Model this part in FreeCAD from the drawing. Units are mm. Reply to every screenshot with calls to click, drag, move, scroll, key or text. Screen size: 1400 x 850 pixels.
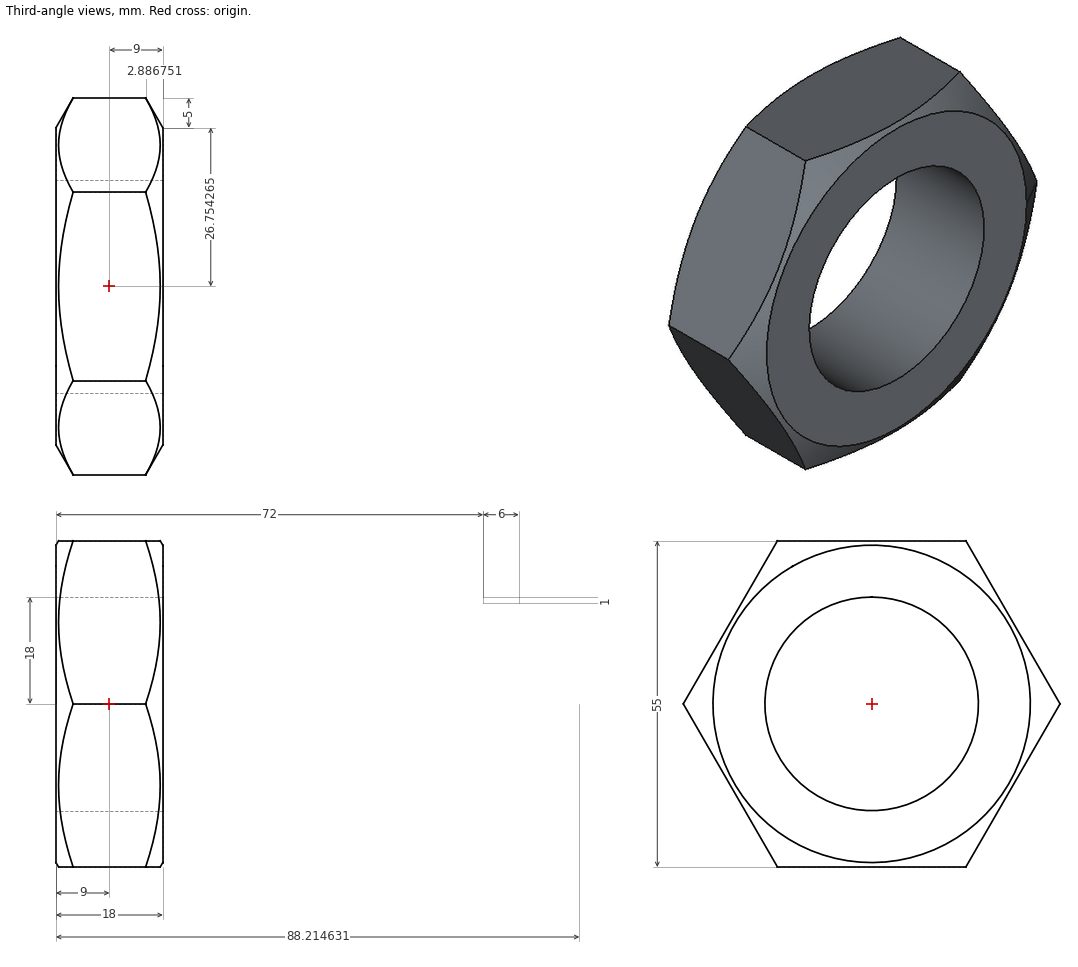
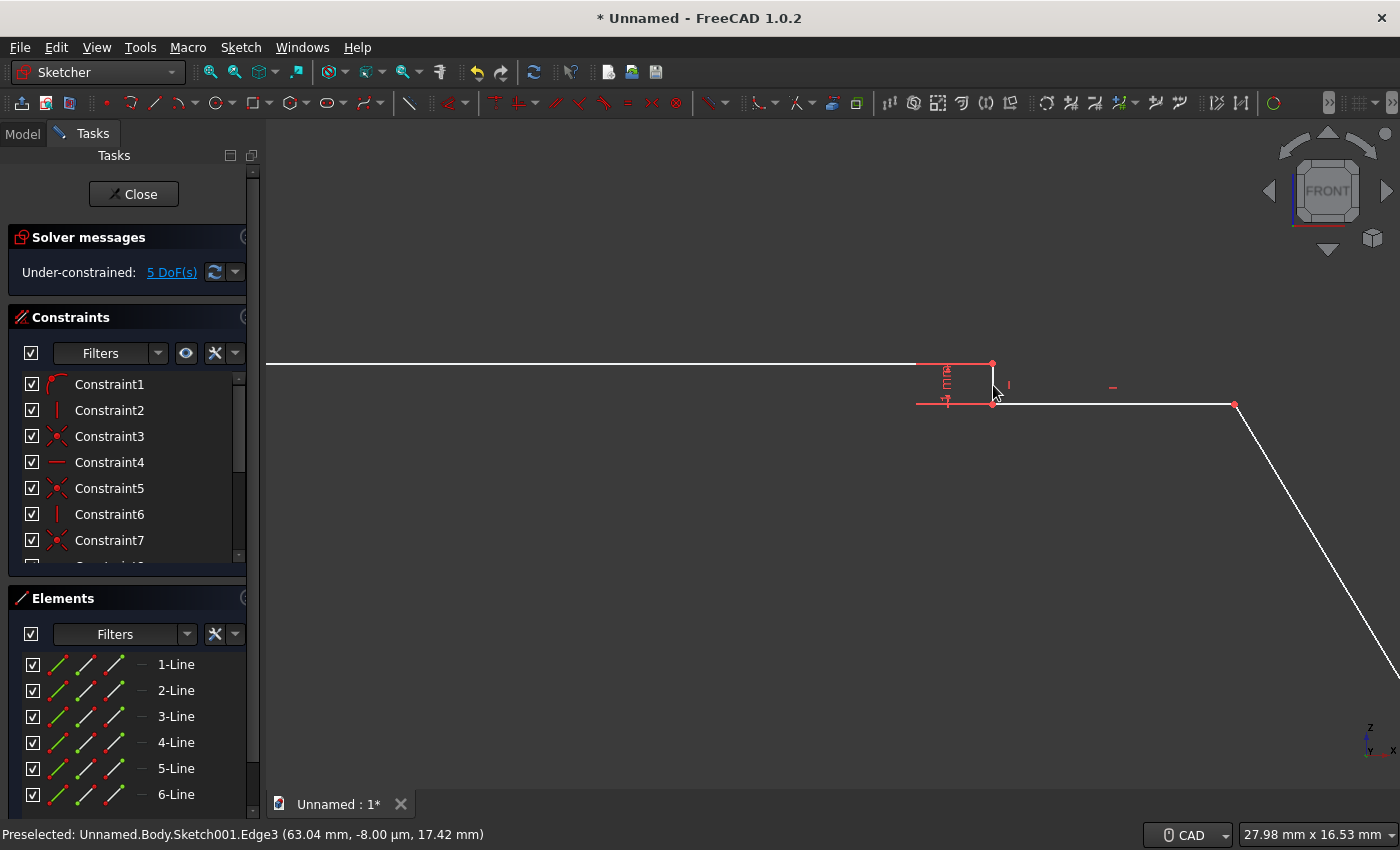
scroll(993, 385, down, 8)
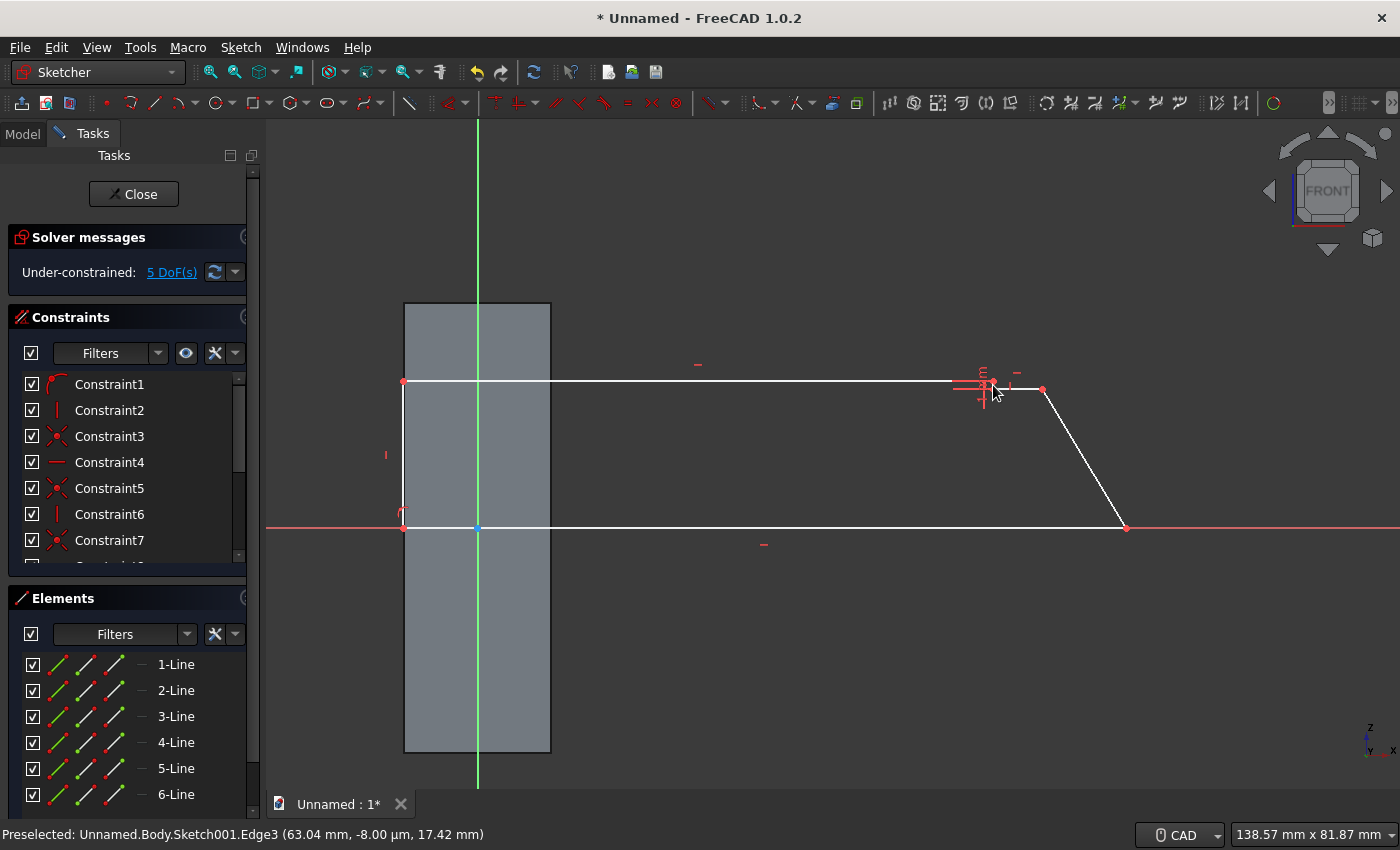
click(1028, 389)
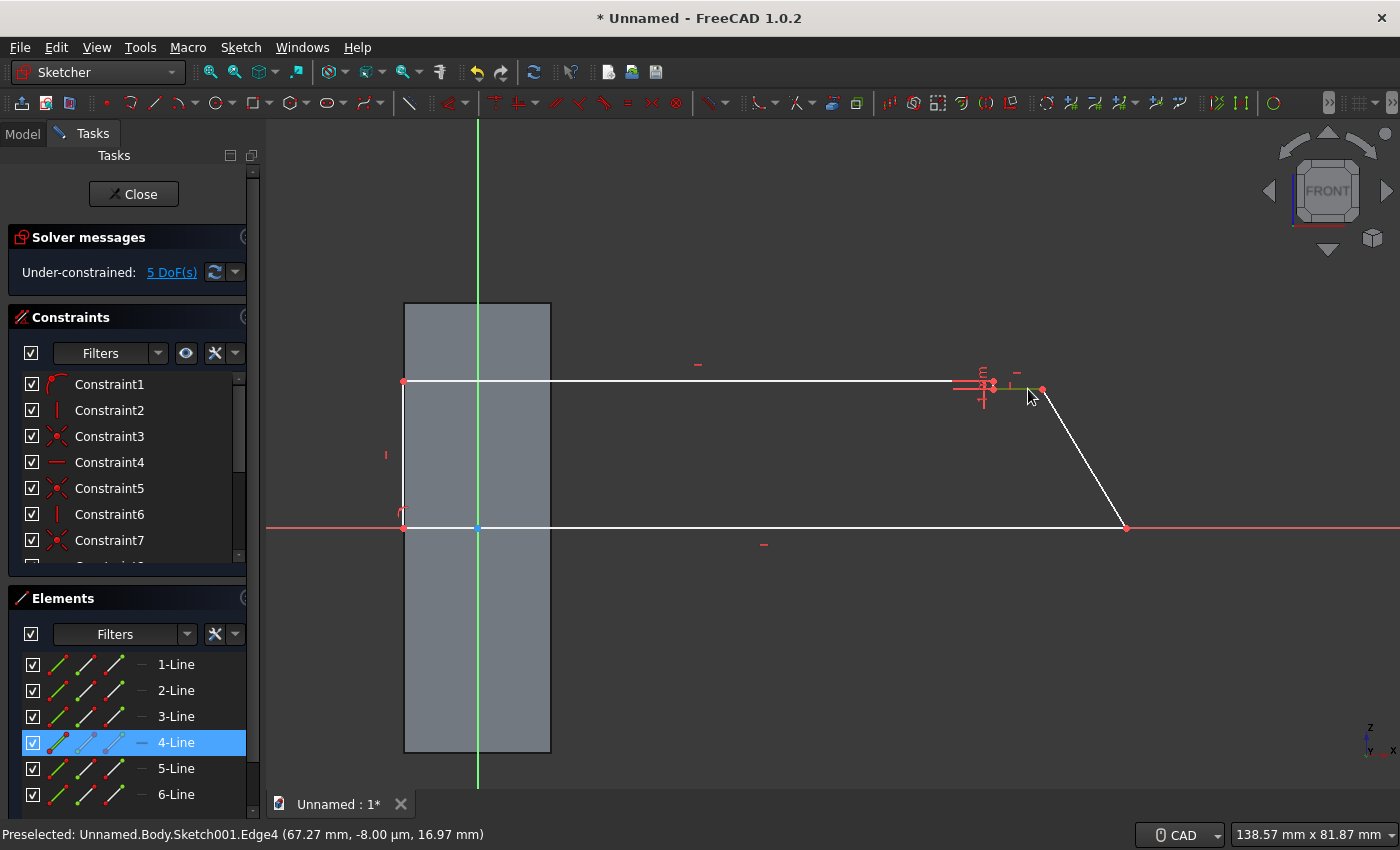
key(l)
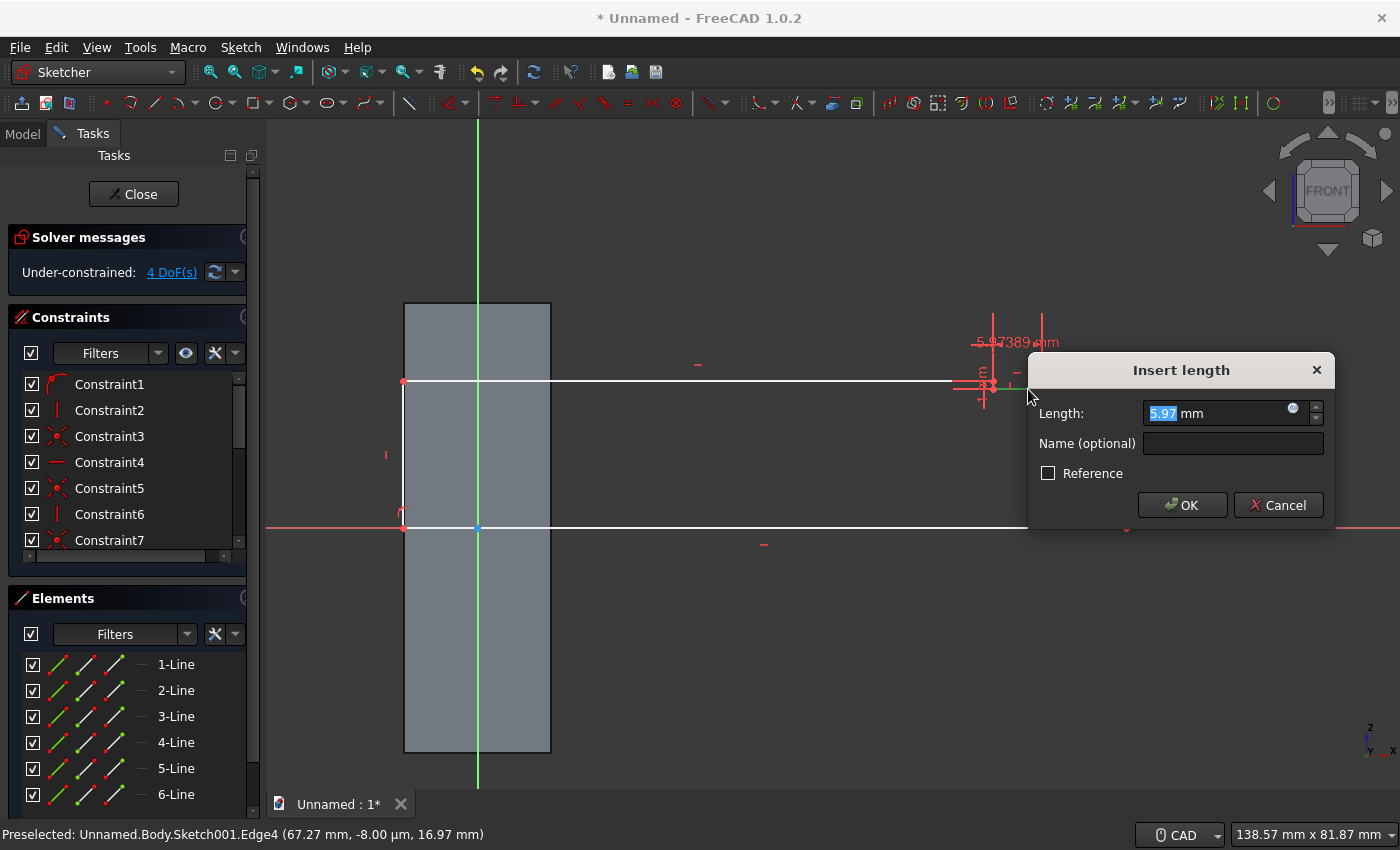
text(6)
key(Return)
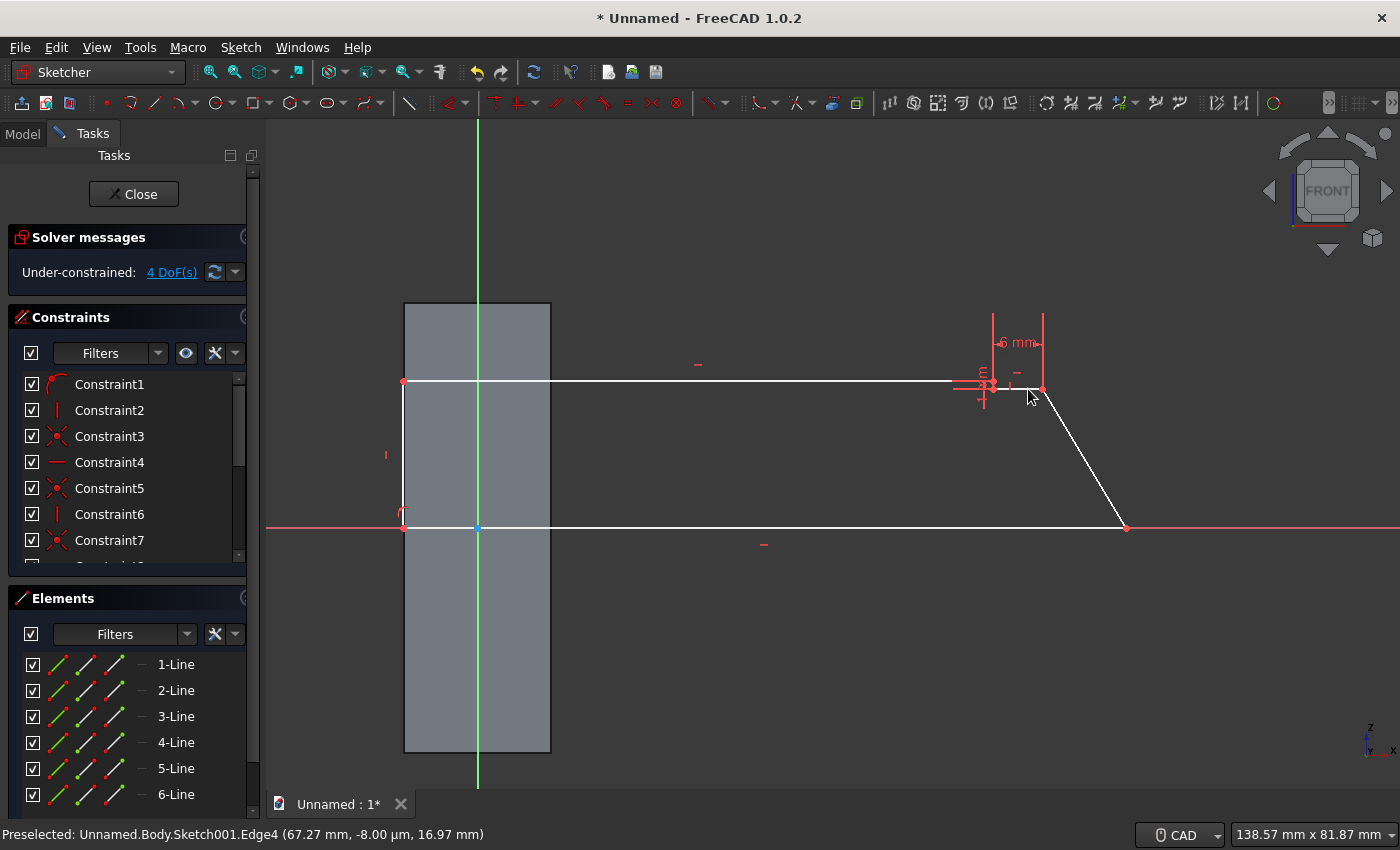
click(403, 484)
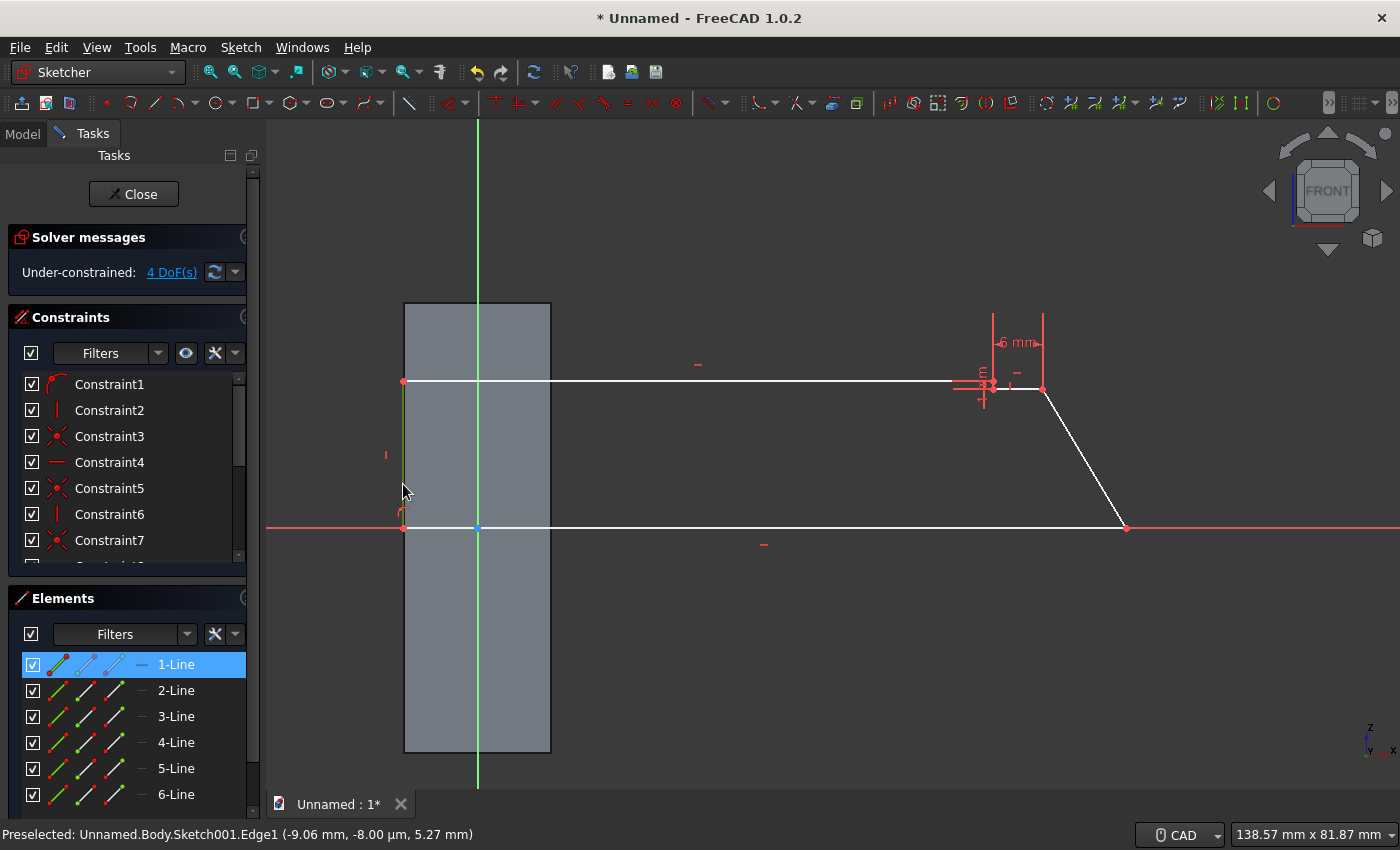
key(i)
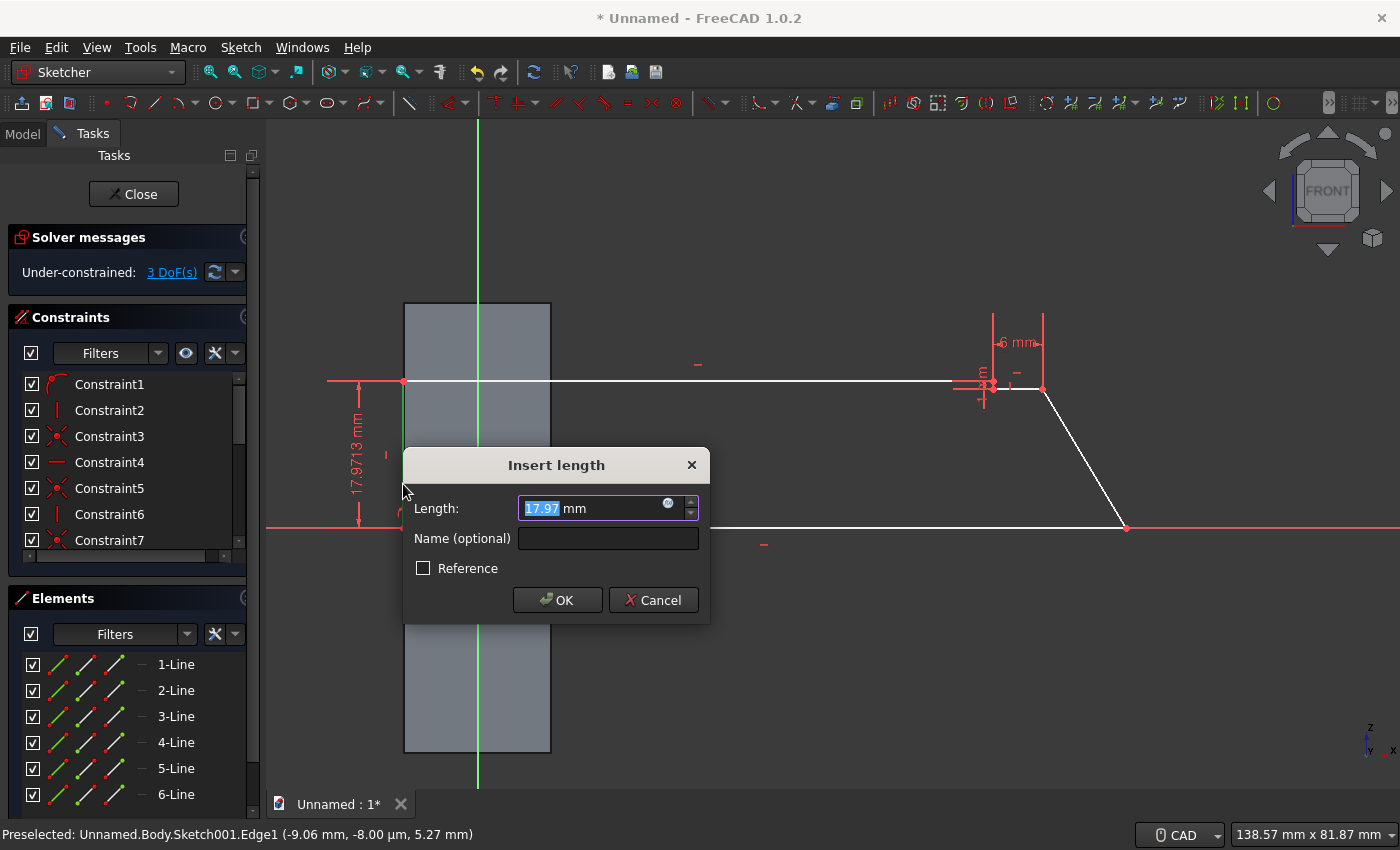
text(18)
key(Return)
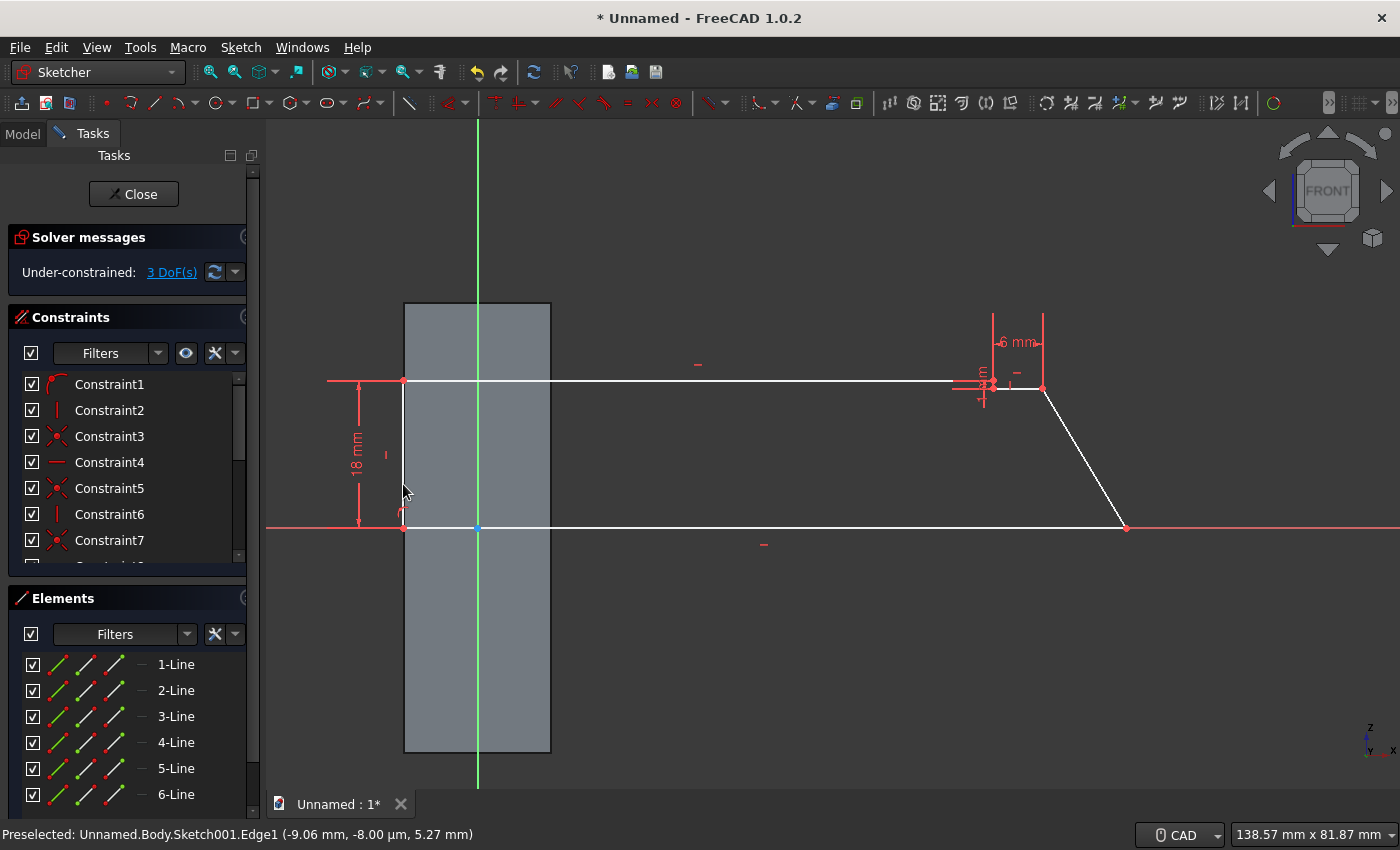
click(580, 381)